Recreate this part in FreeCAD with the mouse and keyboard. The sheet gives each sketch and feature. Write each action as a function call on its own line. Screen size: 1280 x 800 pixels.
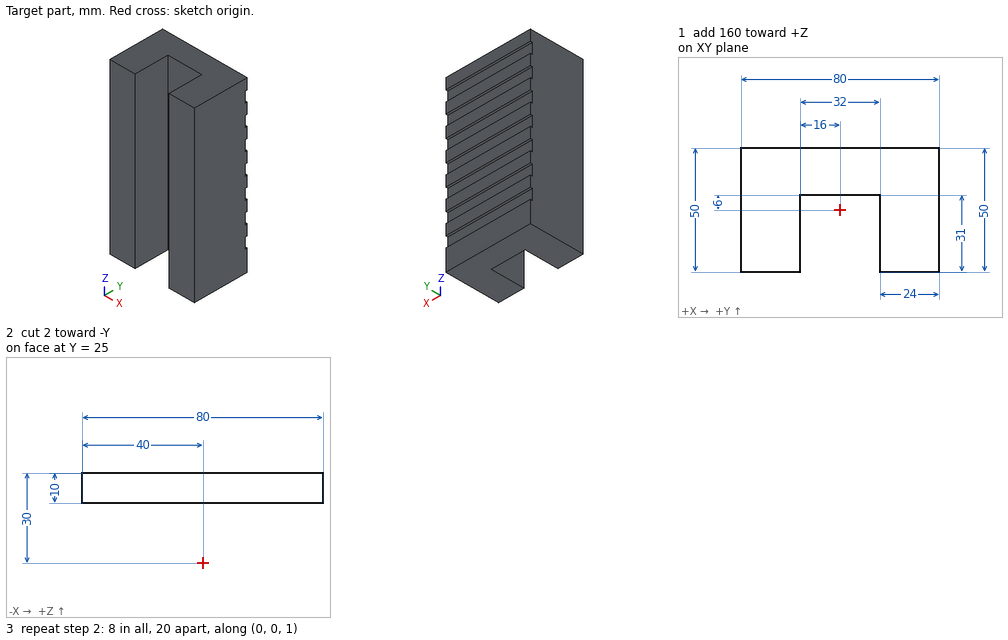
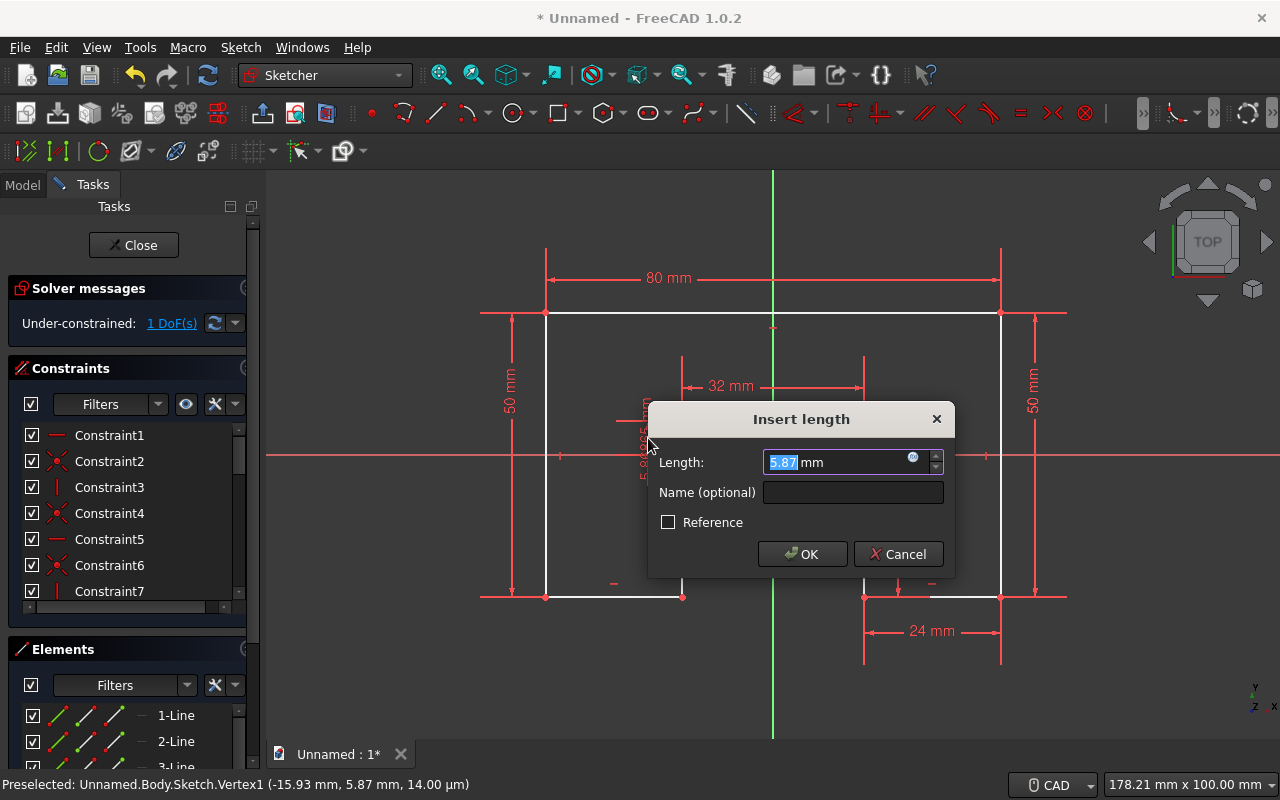
text(6)
key(Return)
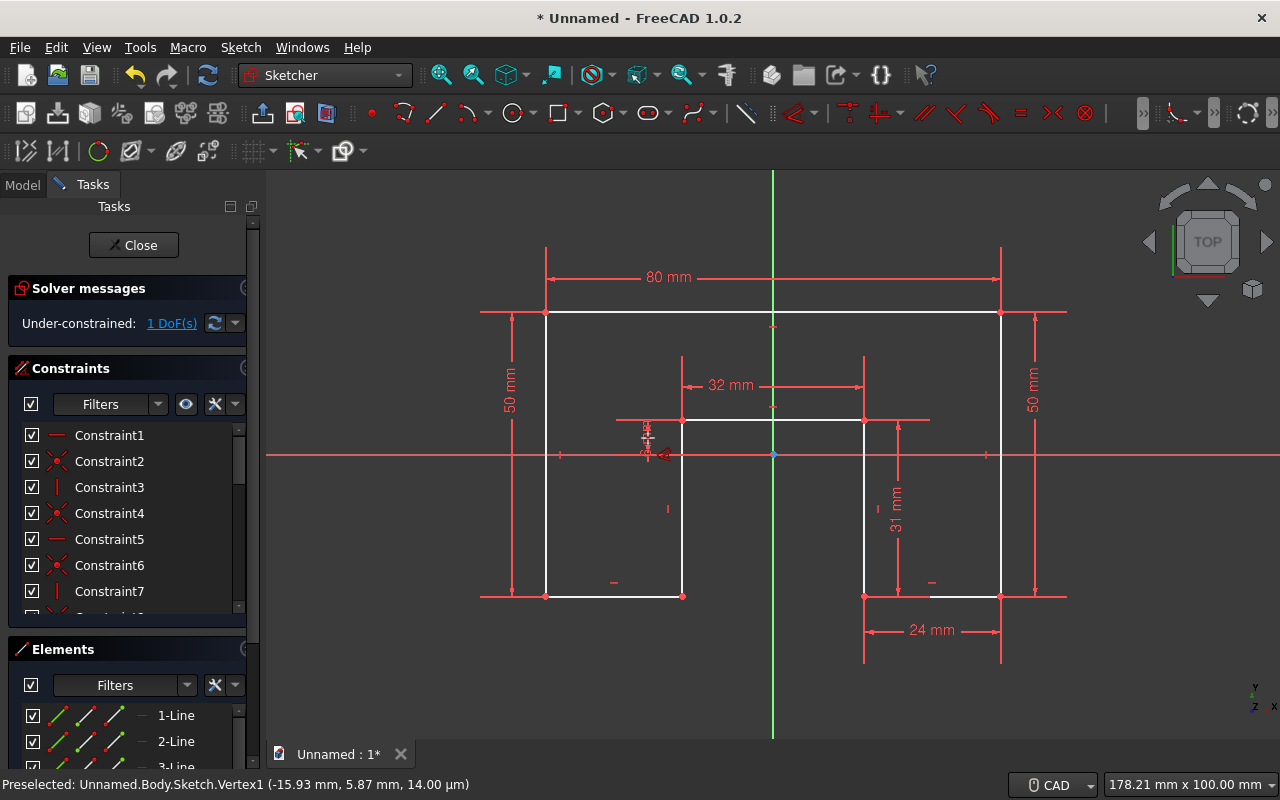
click(682, 420)
click(728, 488)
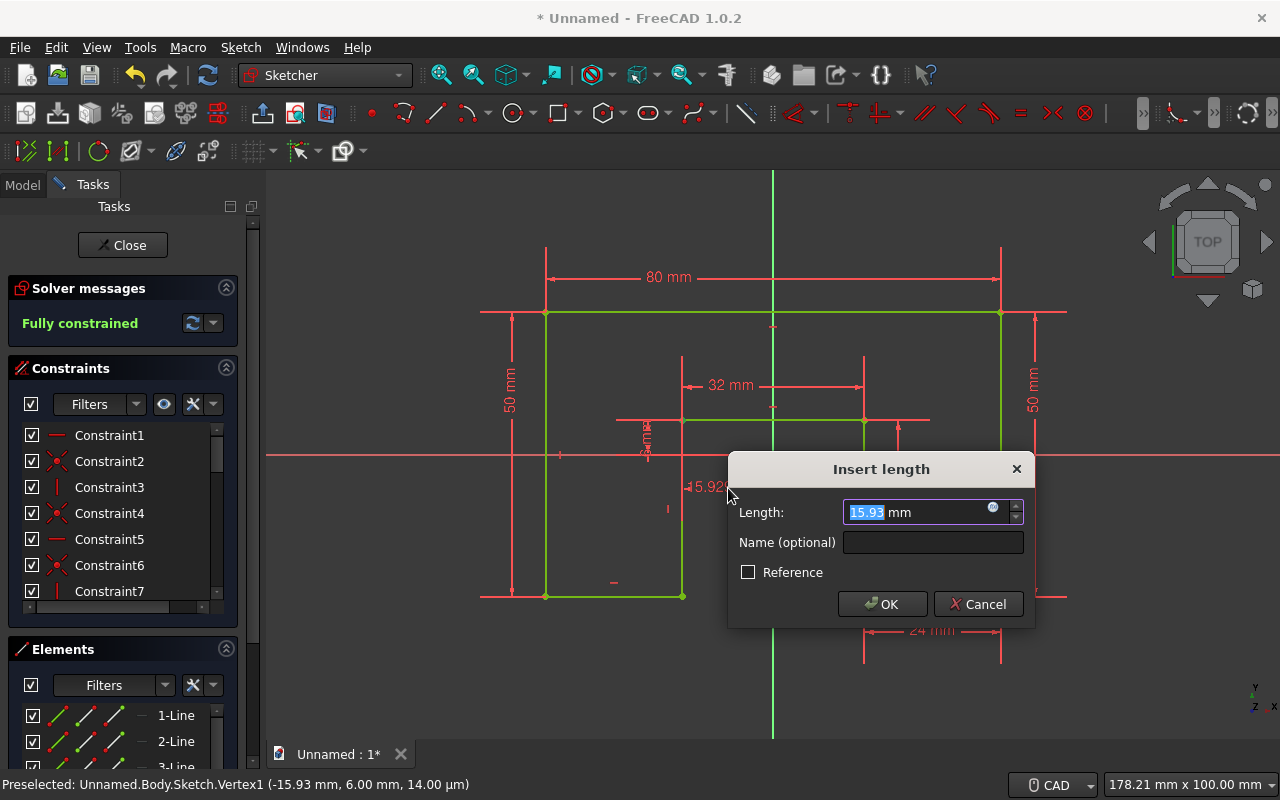
text(16)
key(Return)
key(Escape)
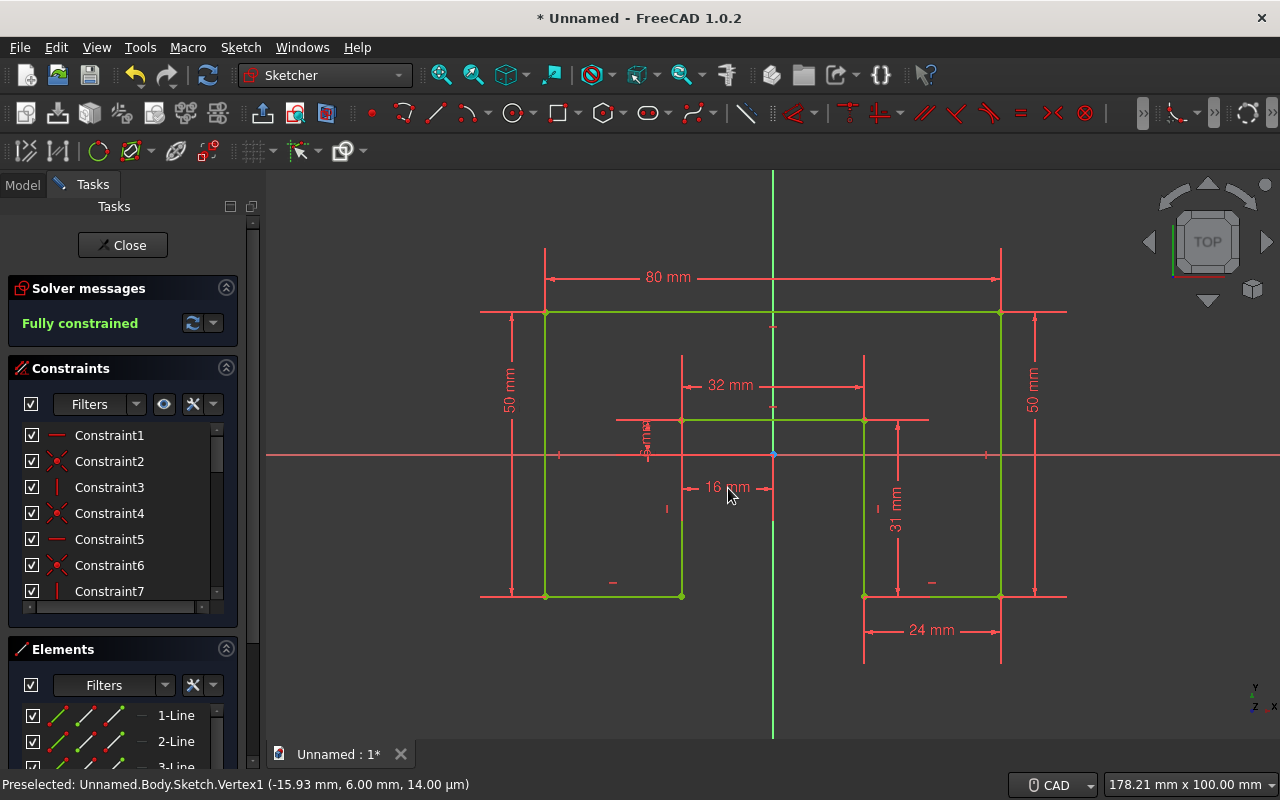
click(123, 245)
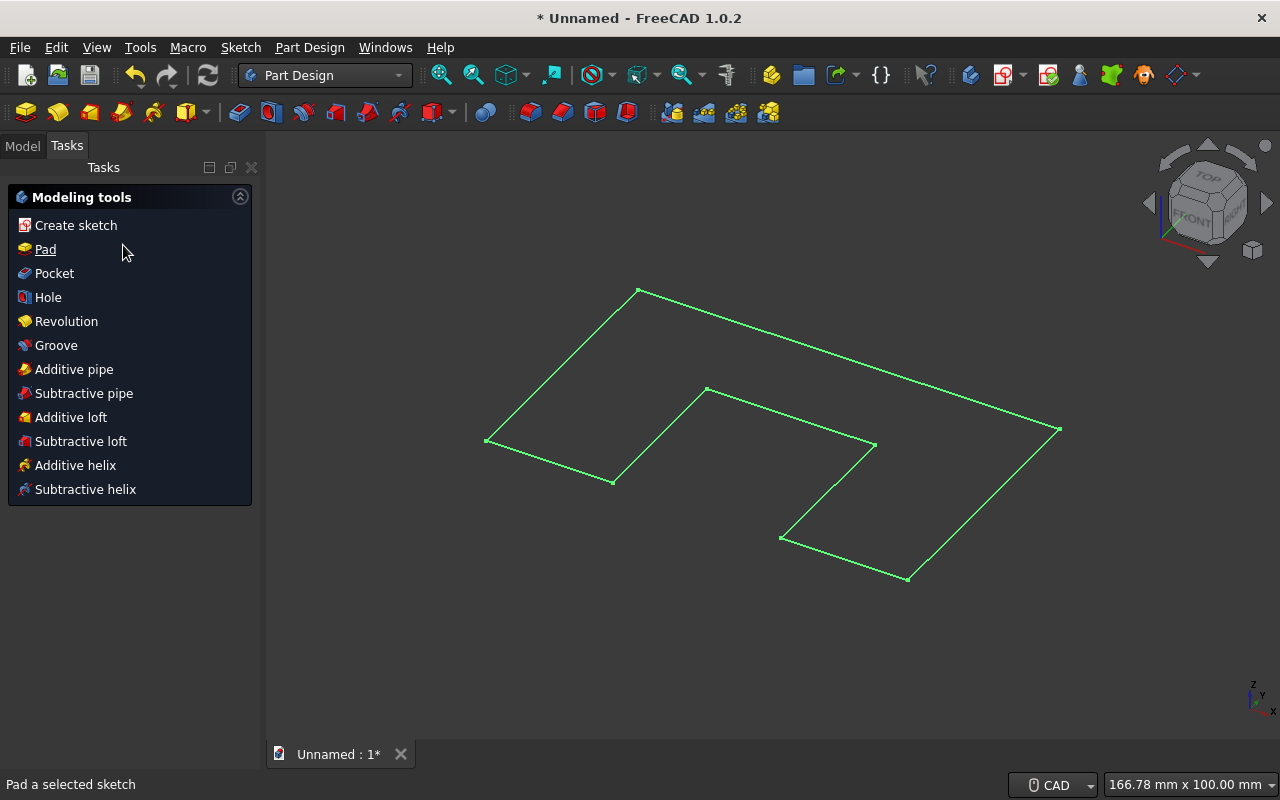
click(26, 112)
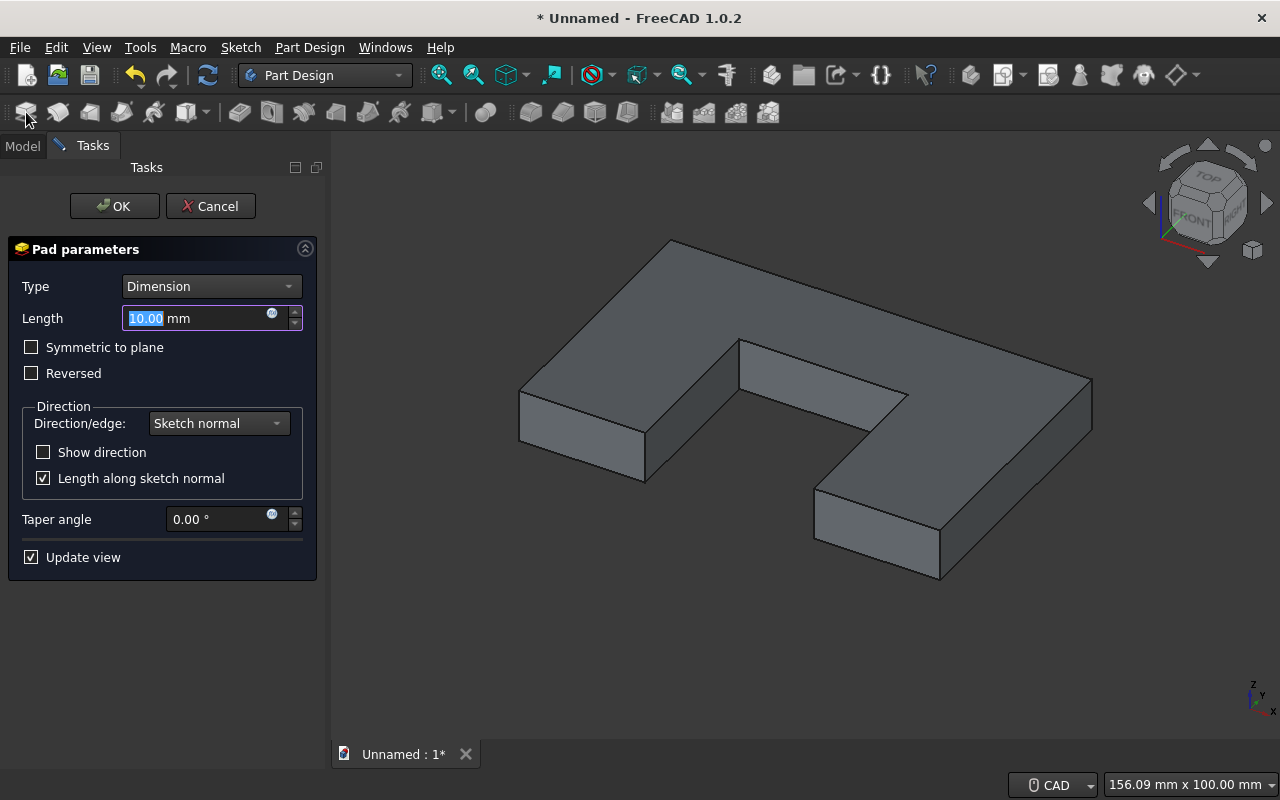
text(160)
key(Tab)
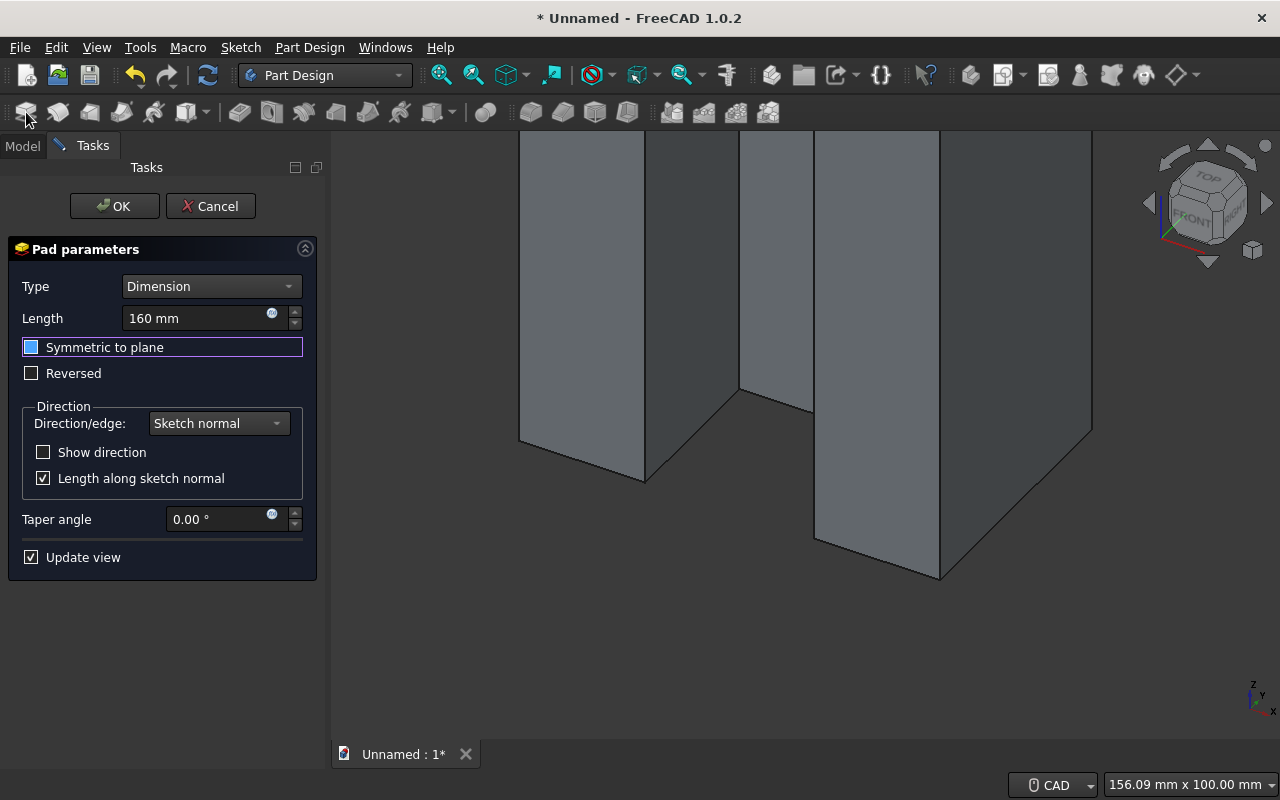
click(115, 206)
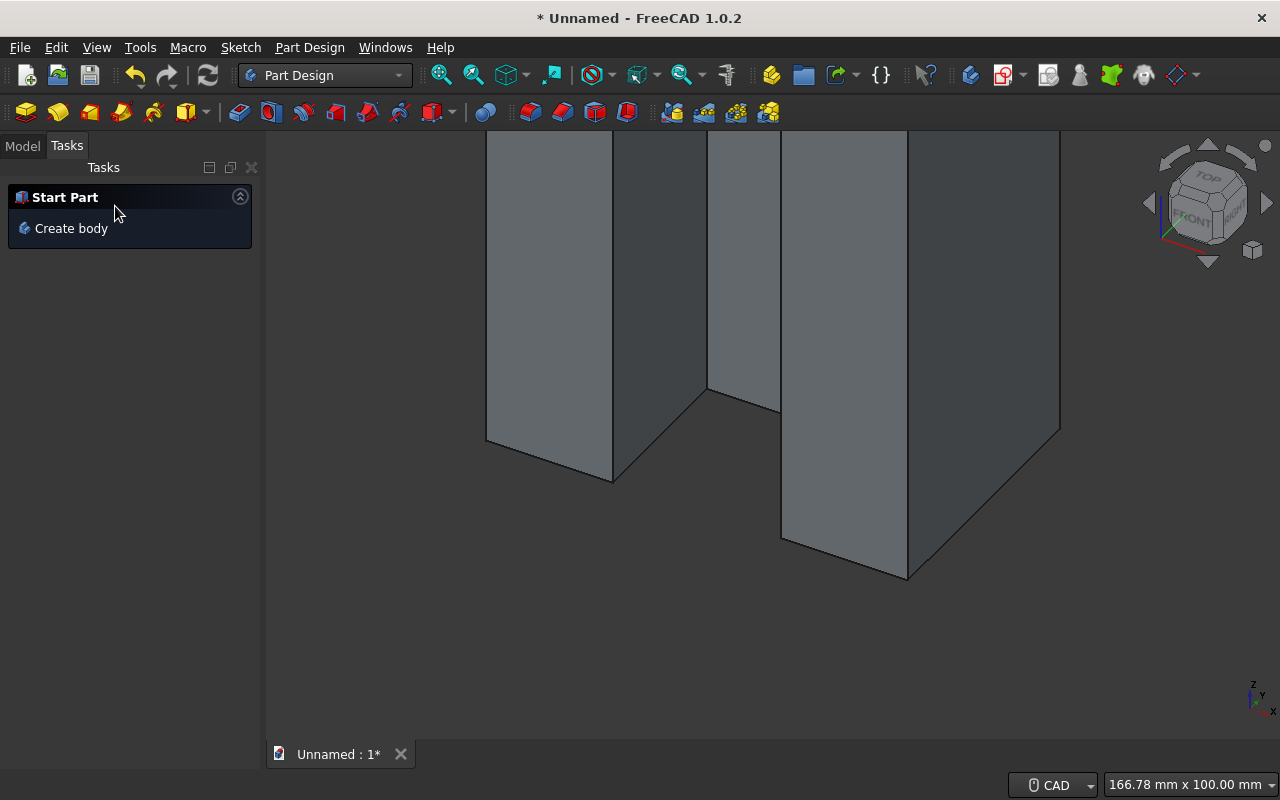
click(442, 76)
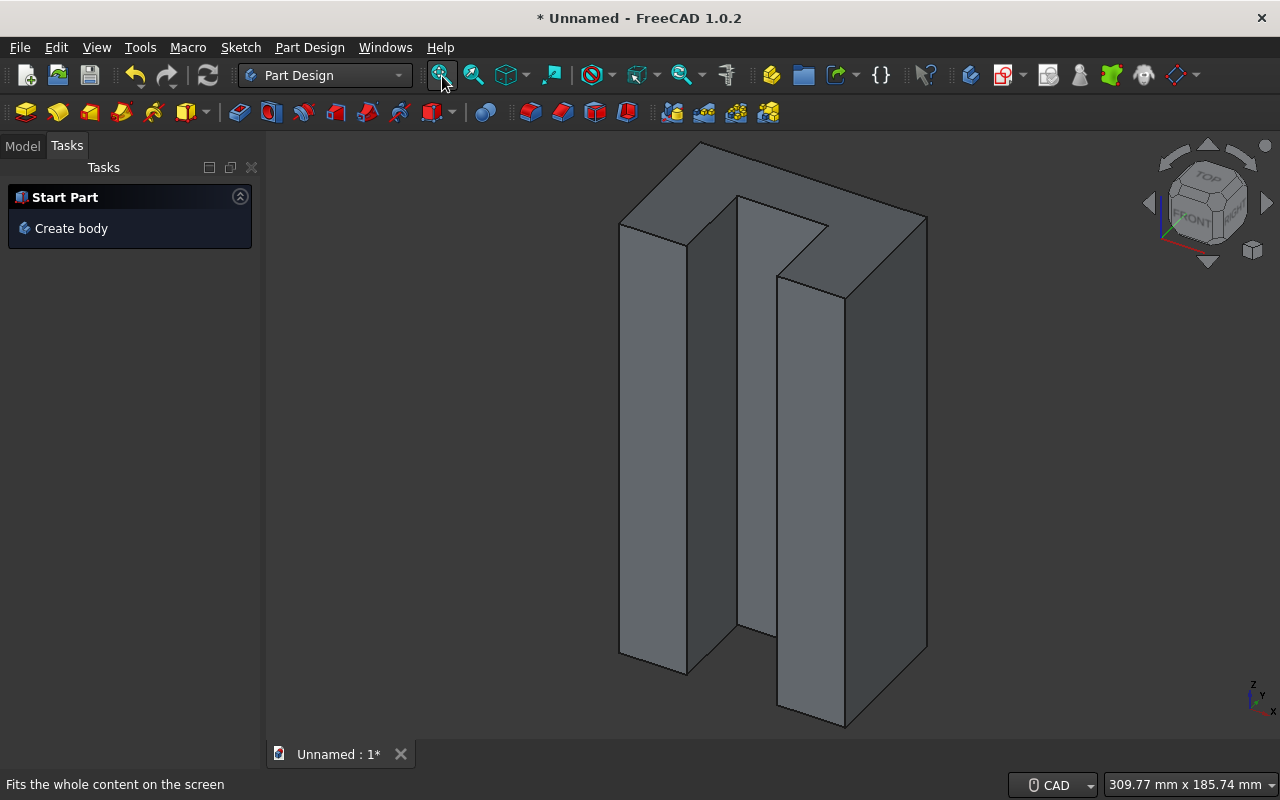
key(4)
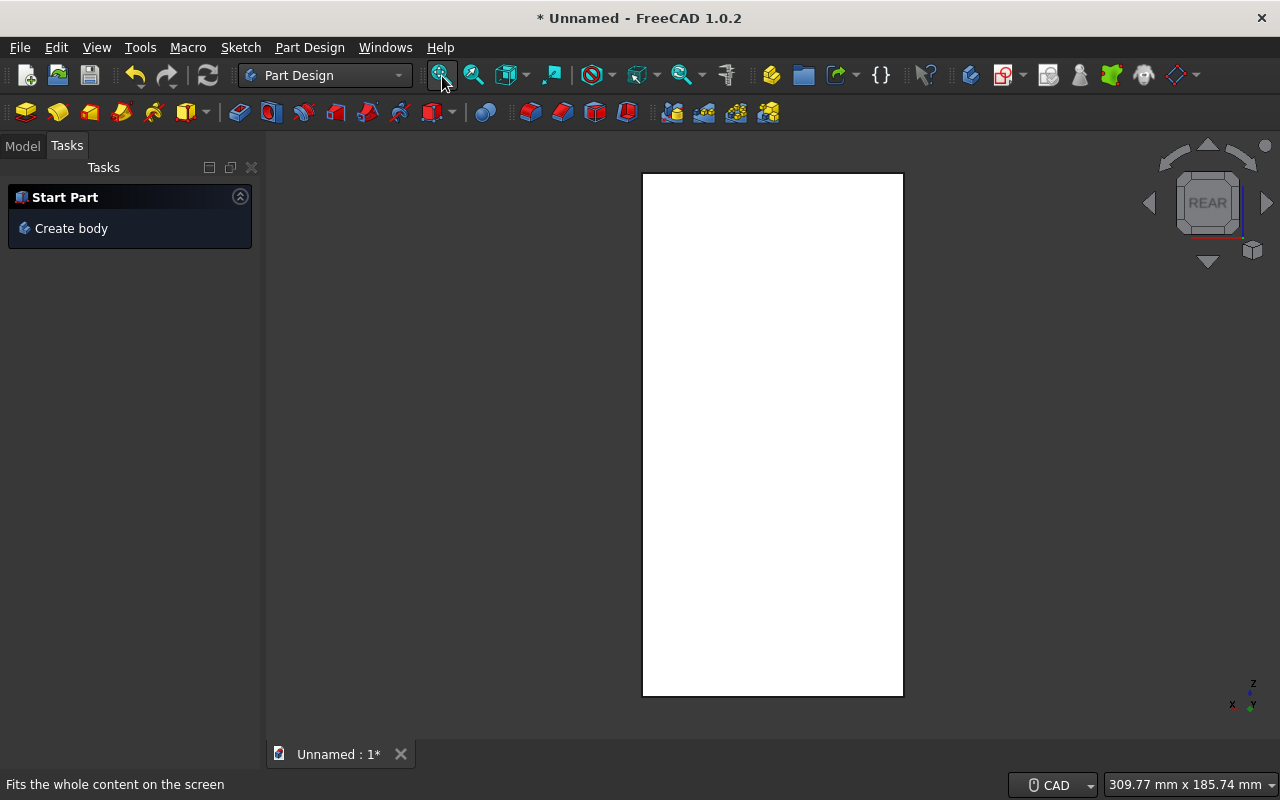
click(773, 359)